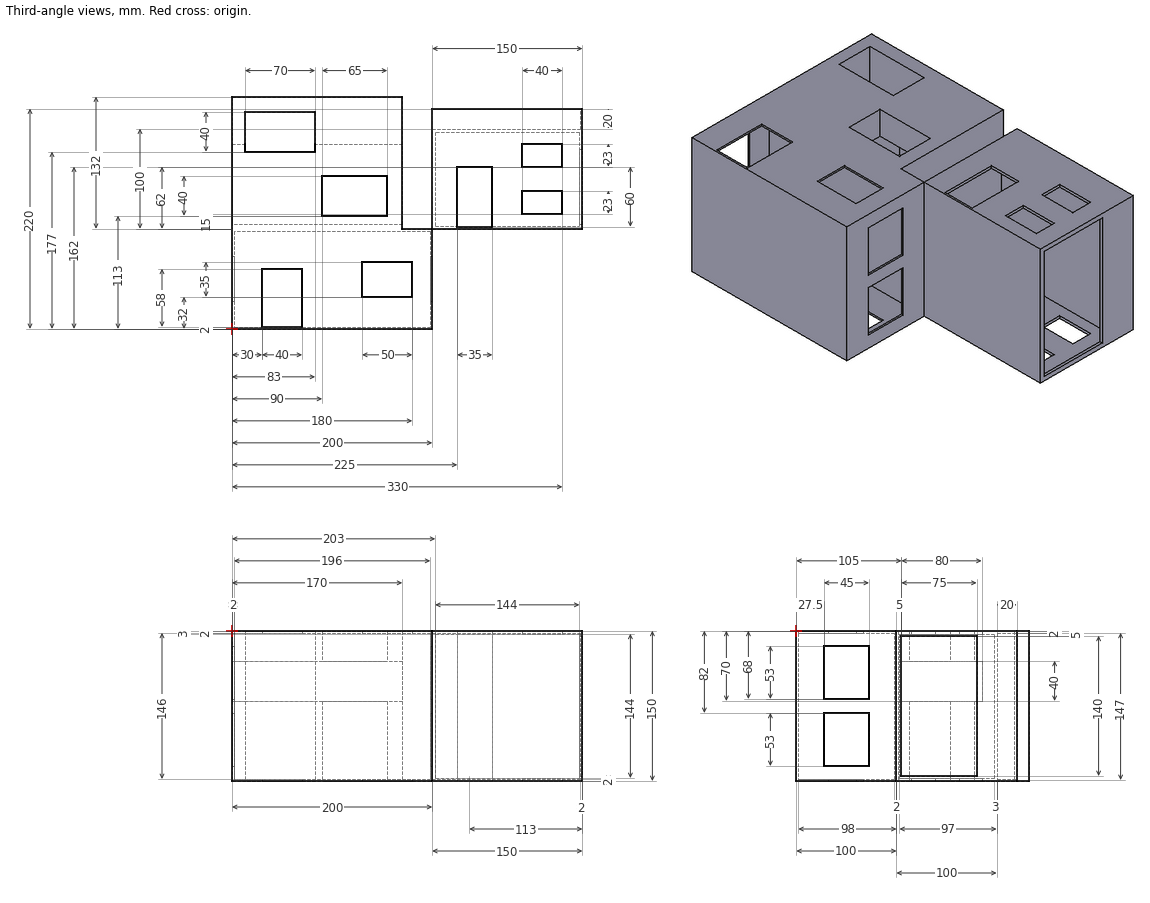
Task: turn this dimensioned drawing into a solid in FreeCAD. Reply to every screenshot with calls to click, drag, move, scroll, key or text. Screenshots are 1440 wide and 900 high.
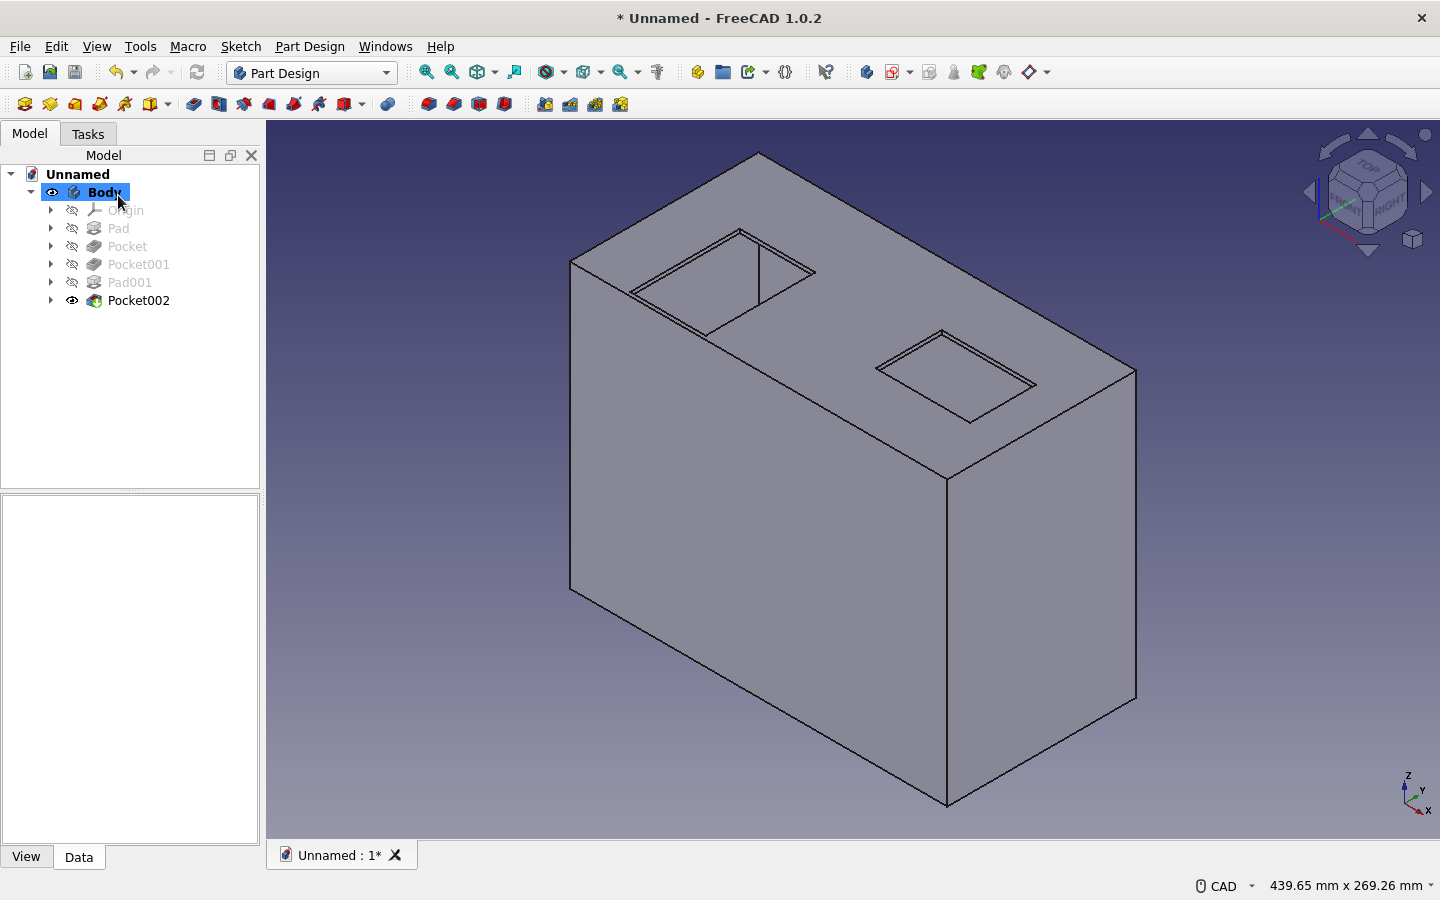
click(1042, 634)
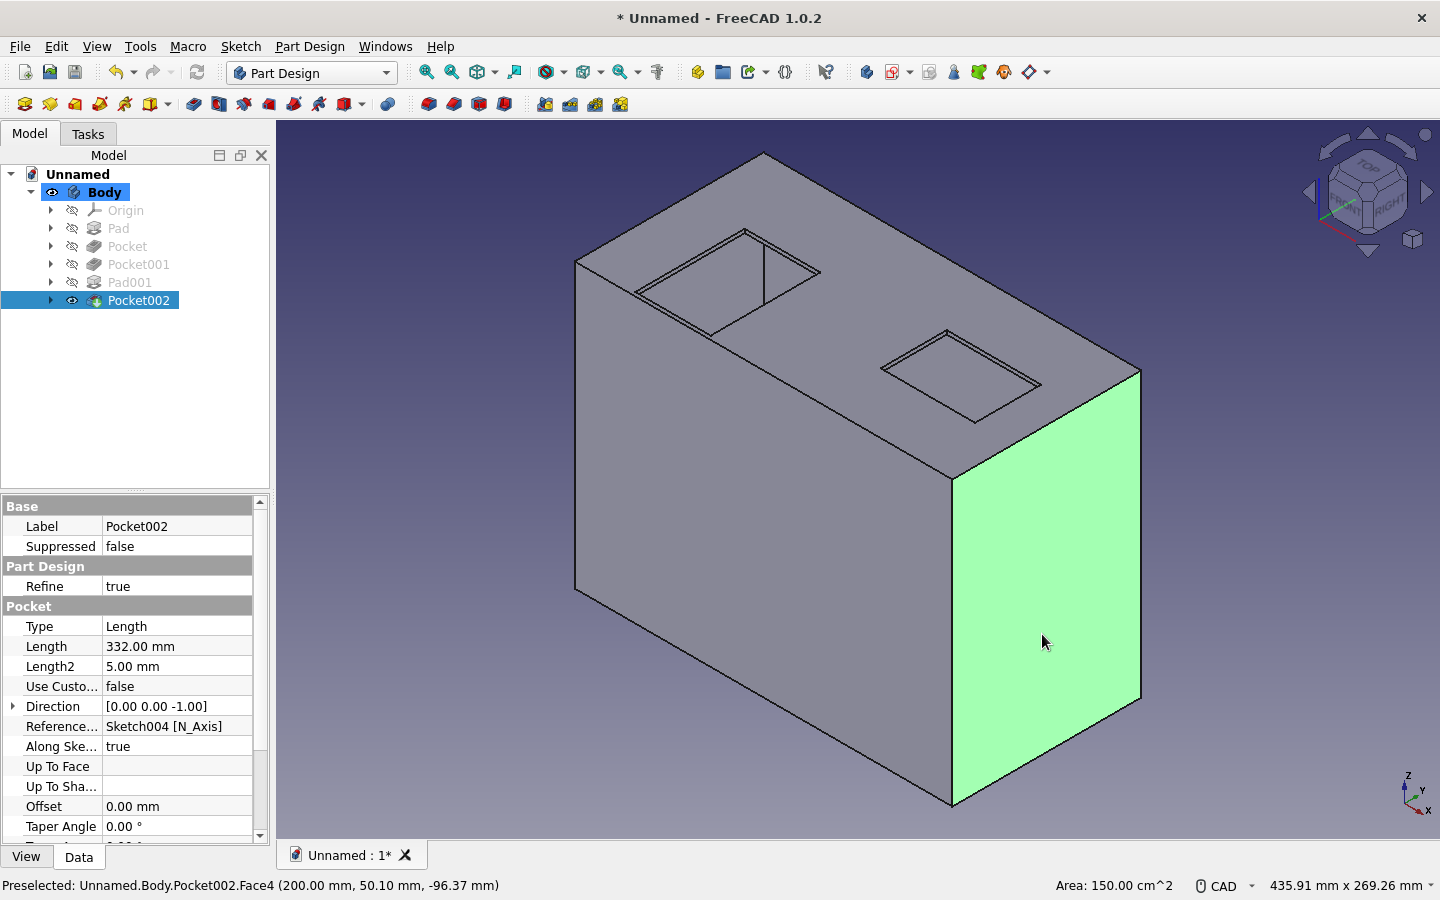
click(892, 72)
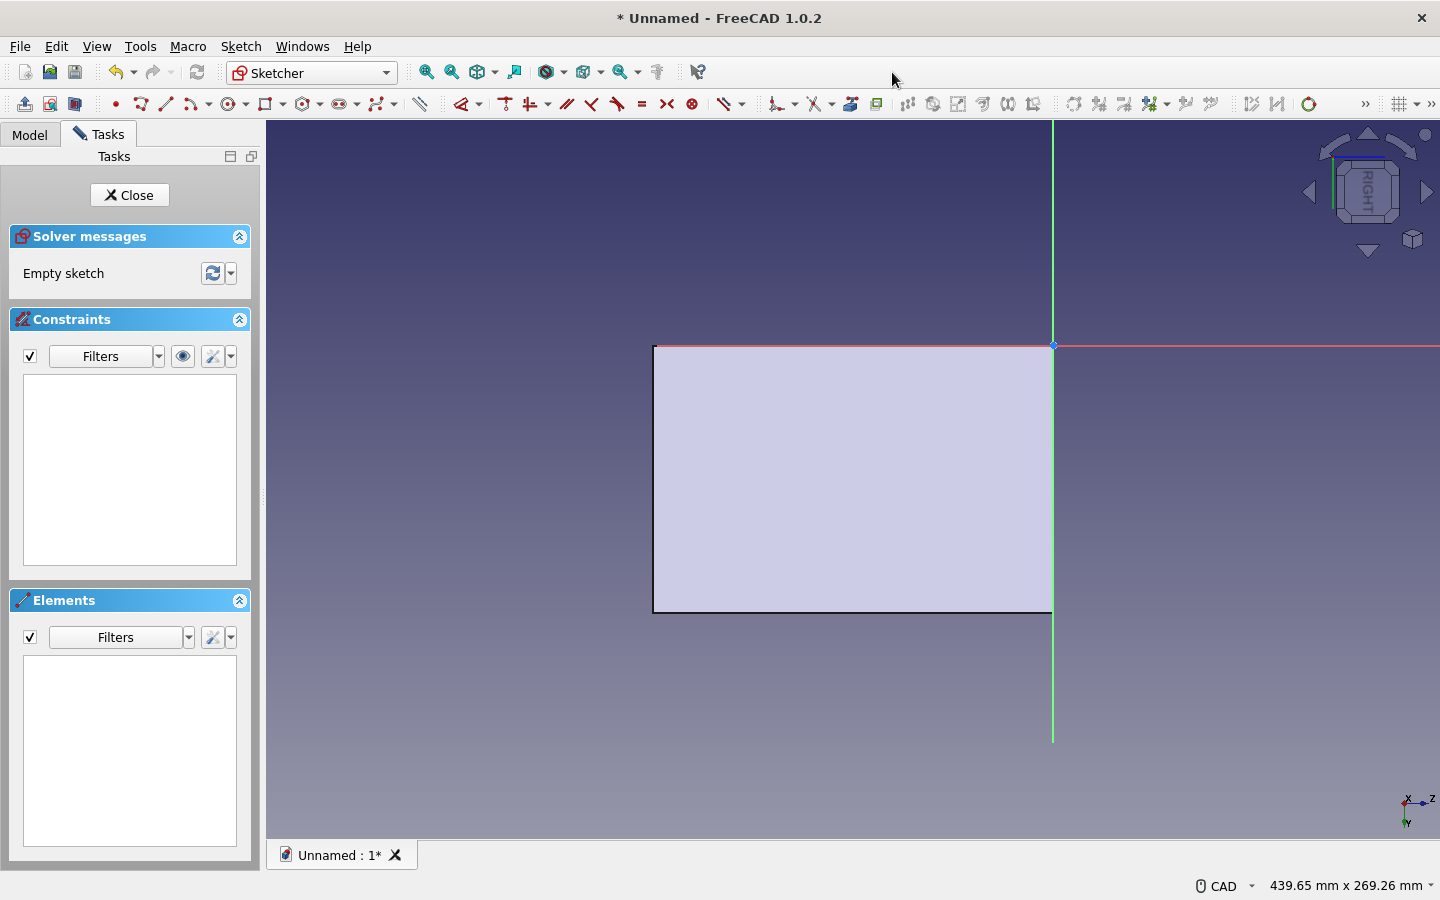
scroll(981, 398, up, 3)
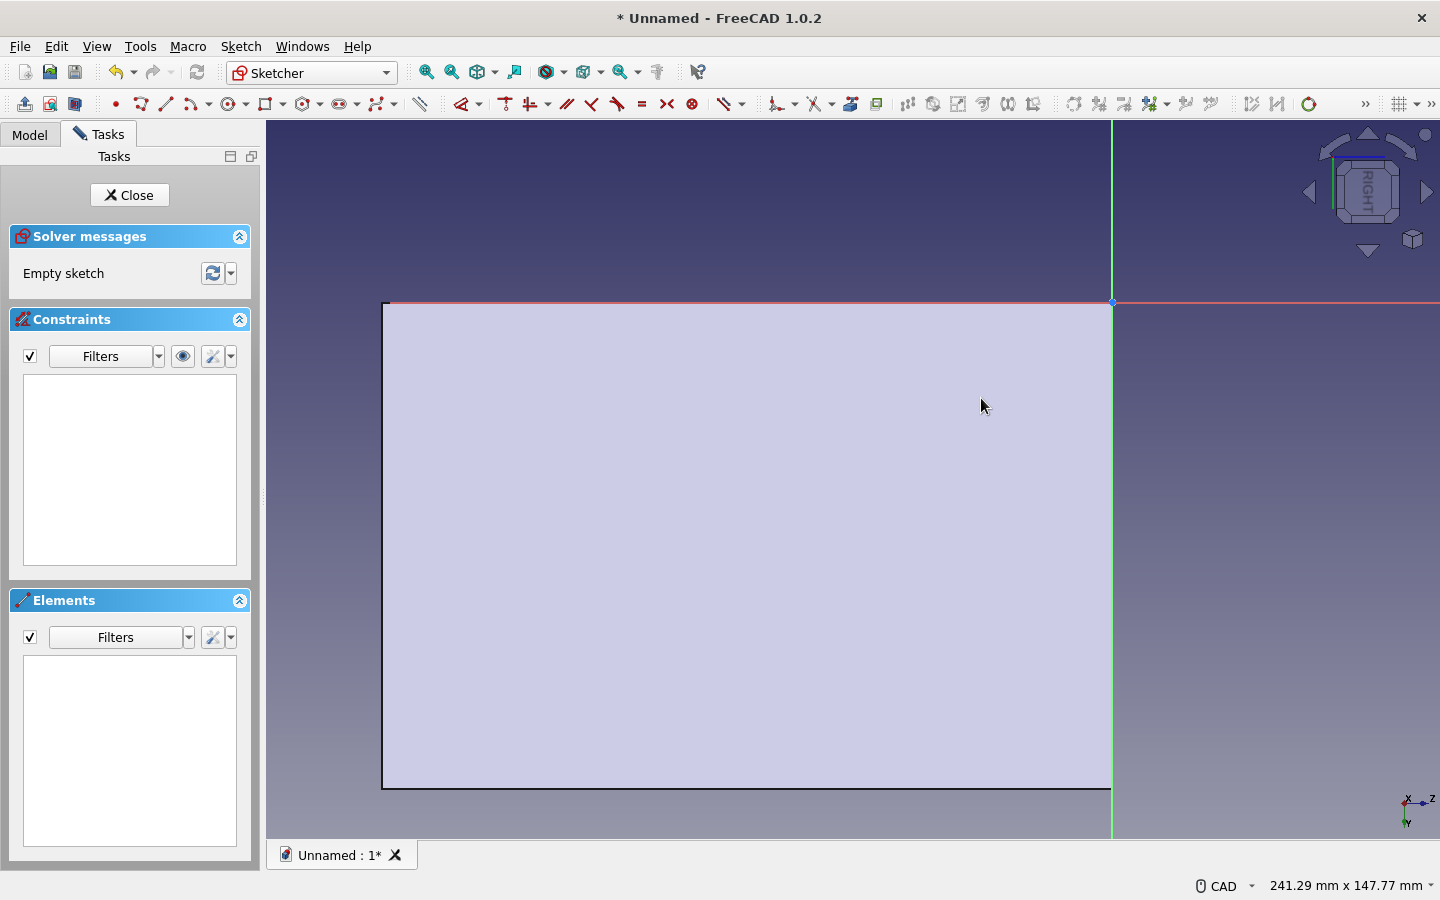
click(264, 104)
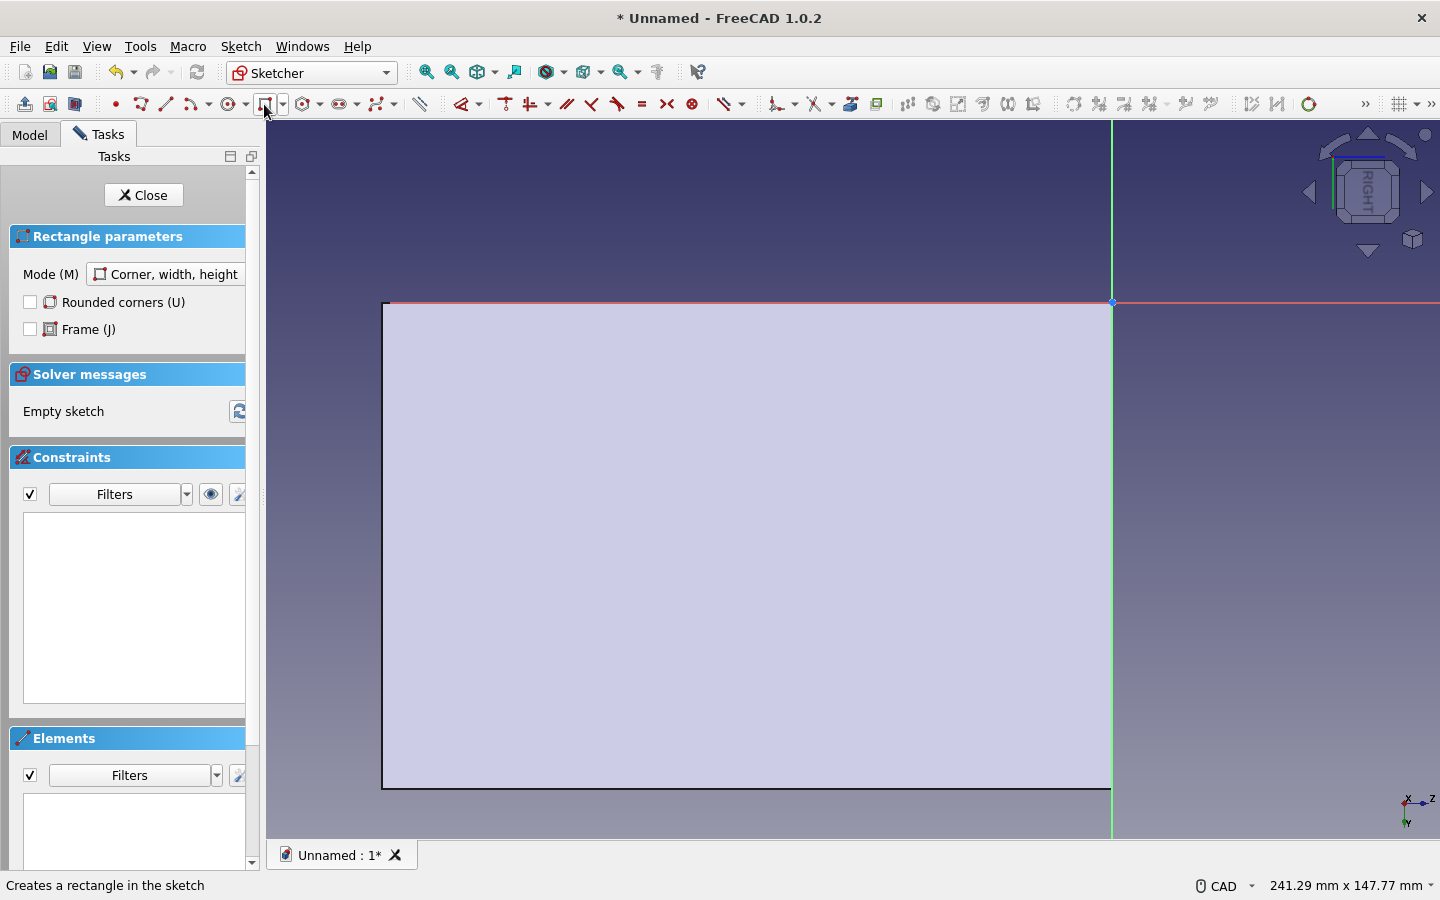
click(781, 437)
move(1039, 656)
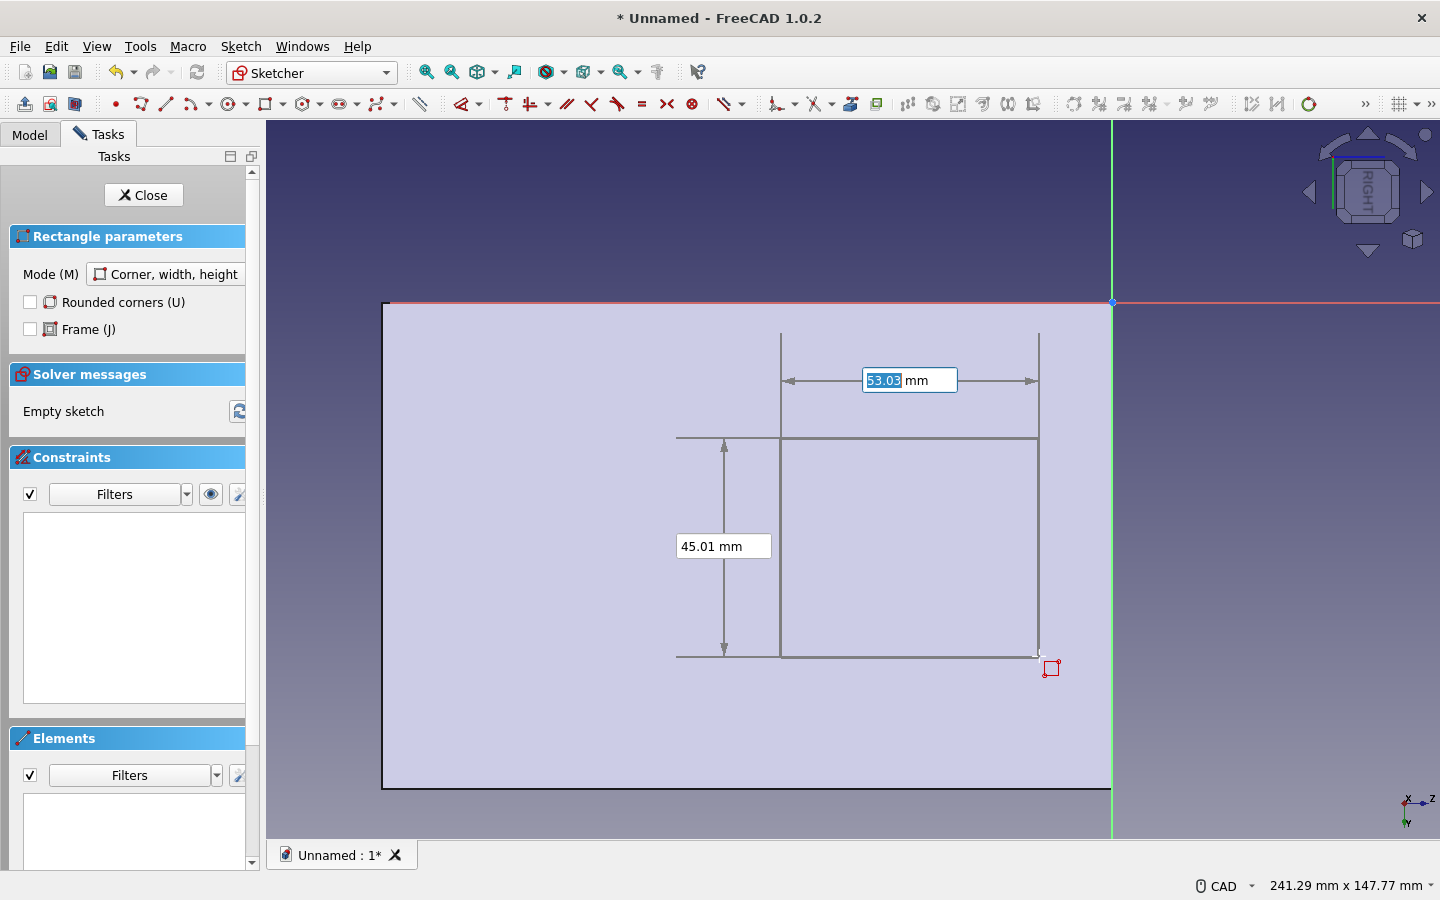
text(53)
key(Tab)
text(45)
key(Return)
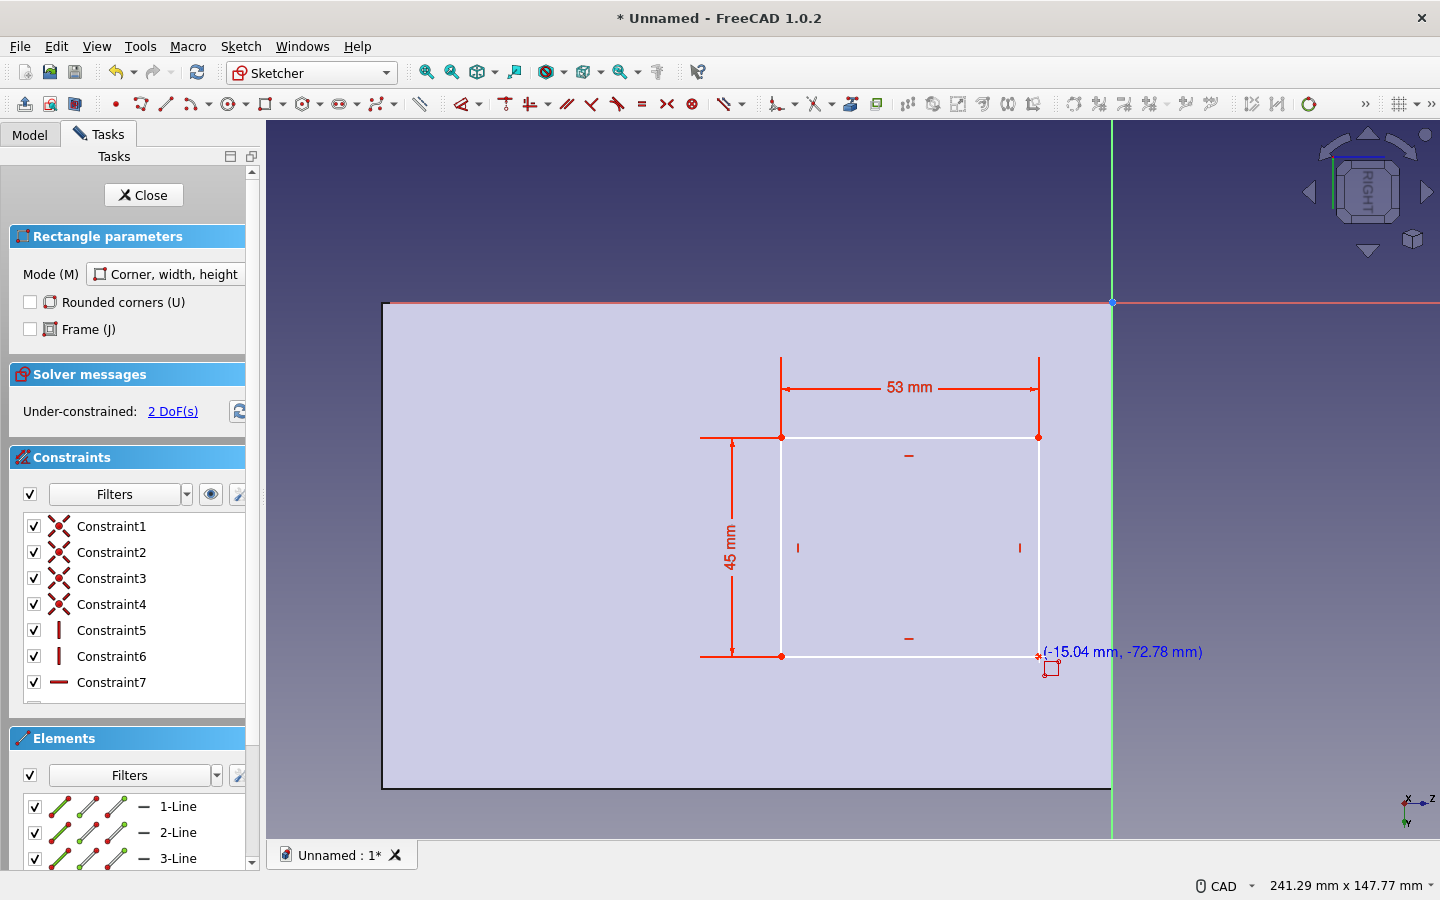
click(455, 437)
move(713, 656)